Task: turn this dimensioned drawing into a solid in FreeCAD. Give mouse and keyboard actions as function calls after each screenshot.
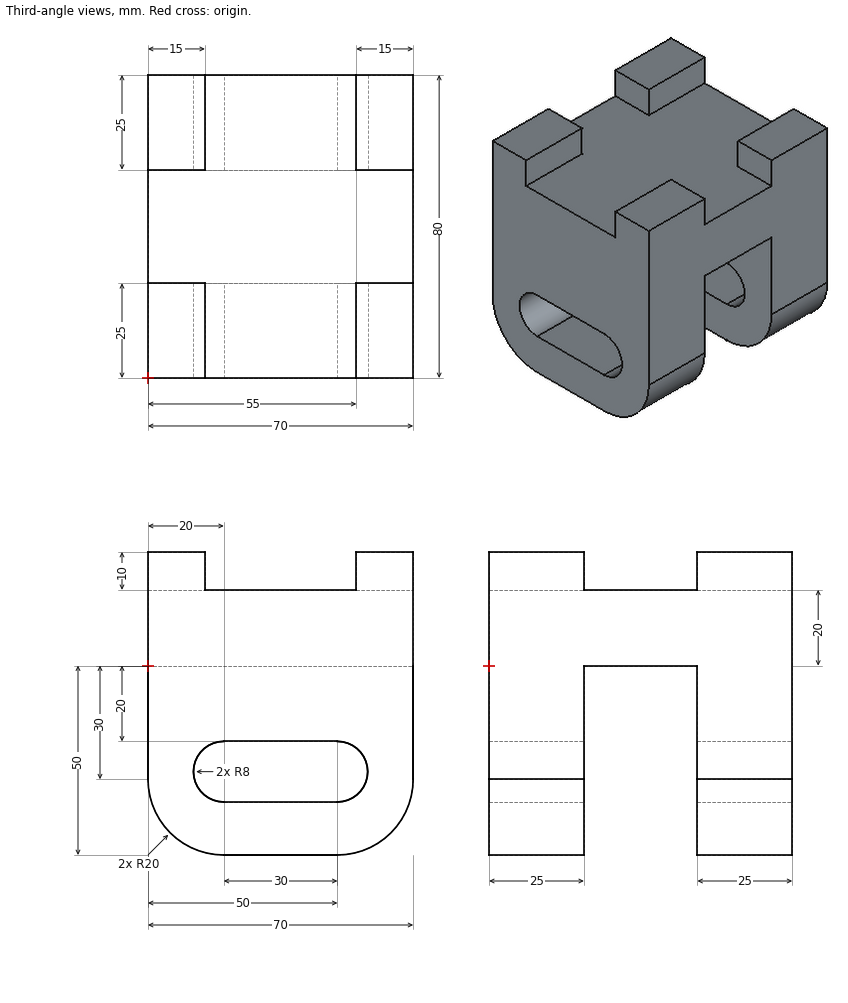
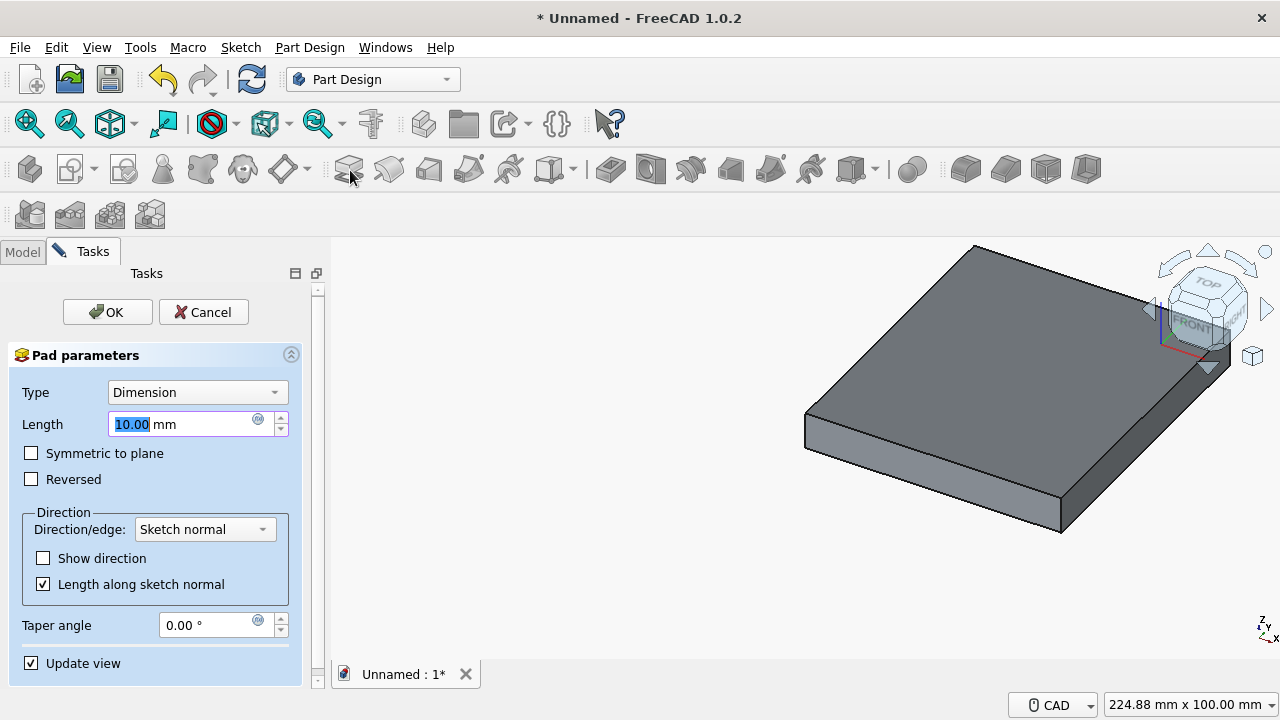
text(20)
key(Tab)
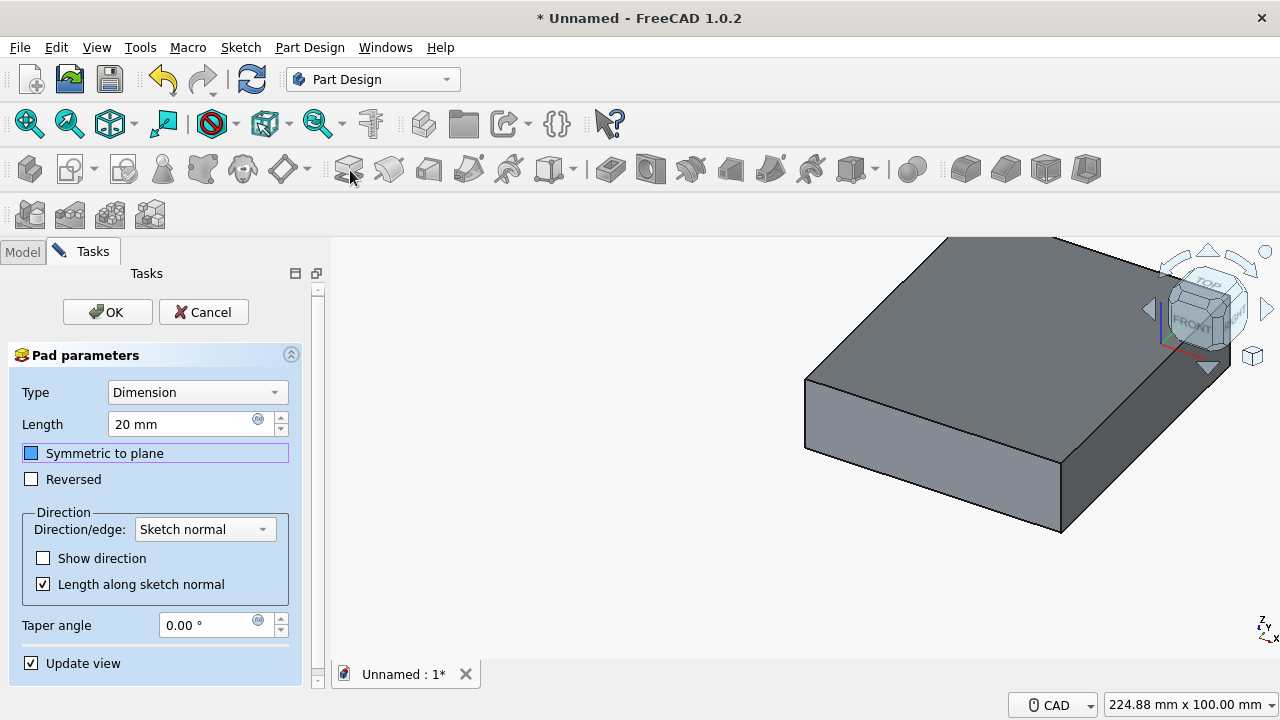
click(108, 312)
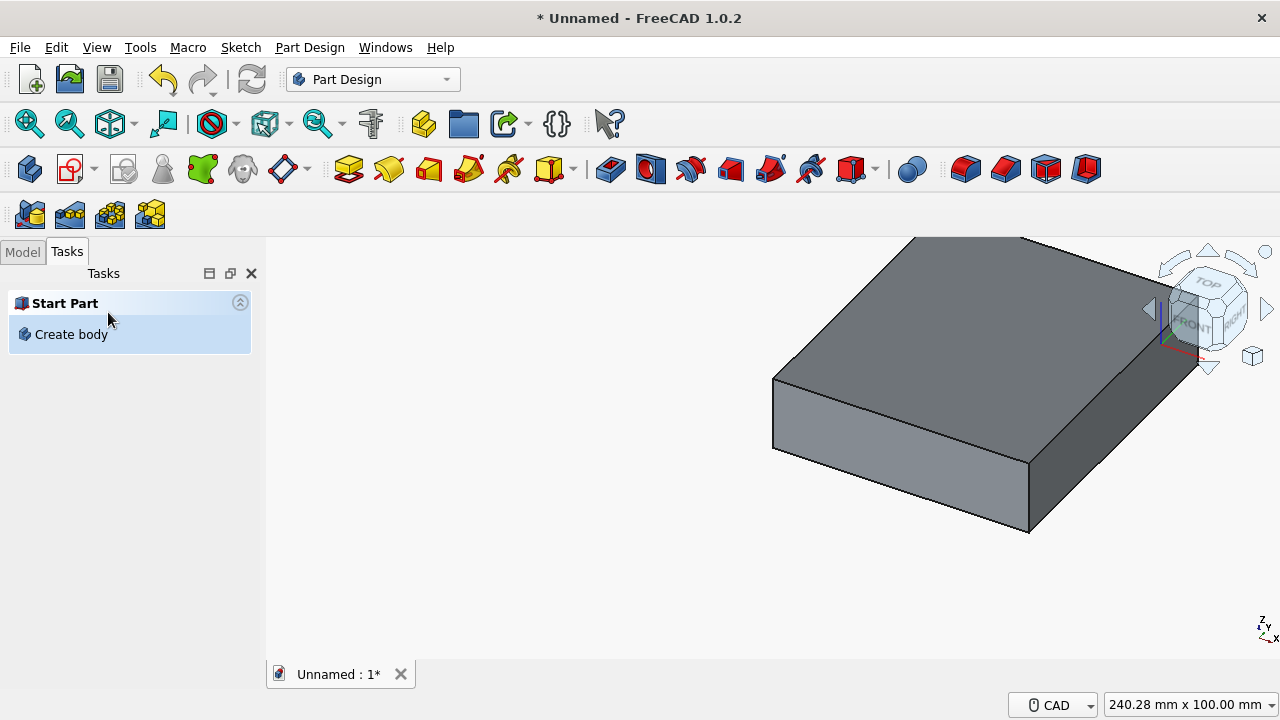
click(30, 124)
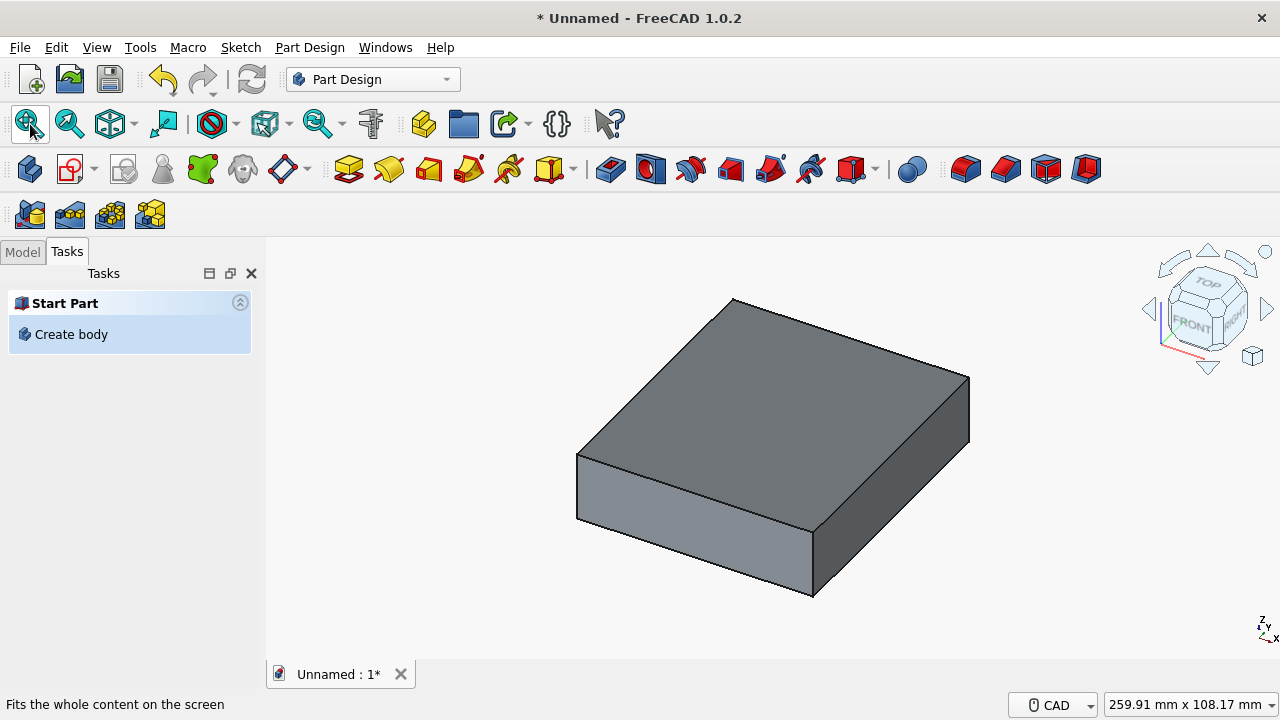
click(773, 415)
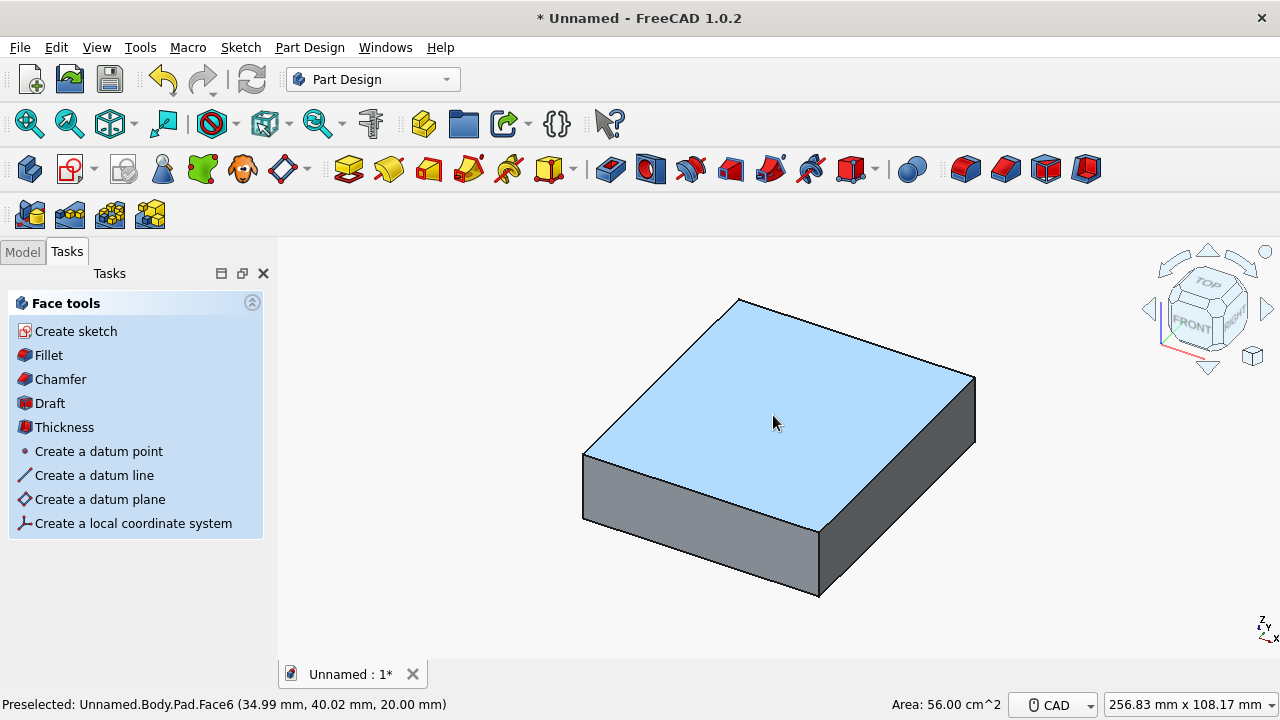
click(70, 170)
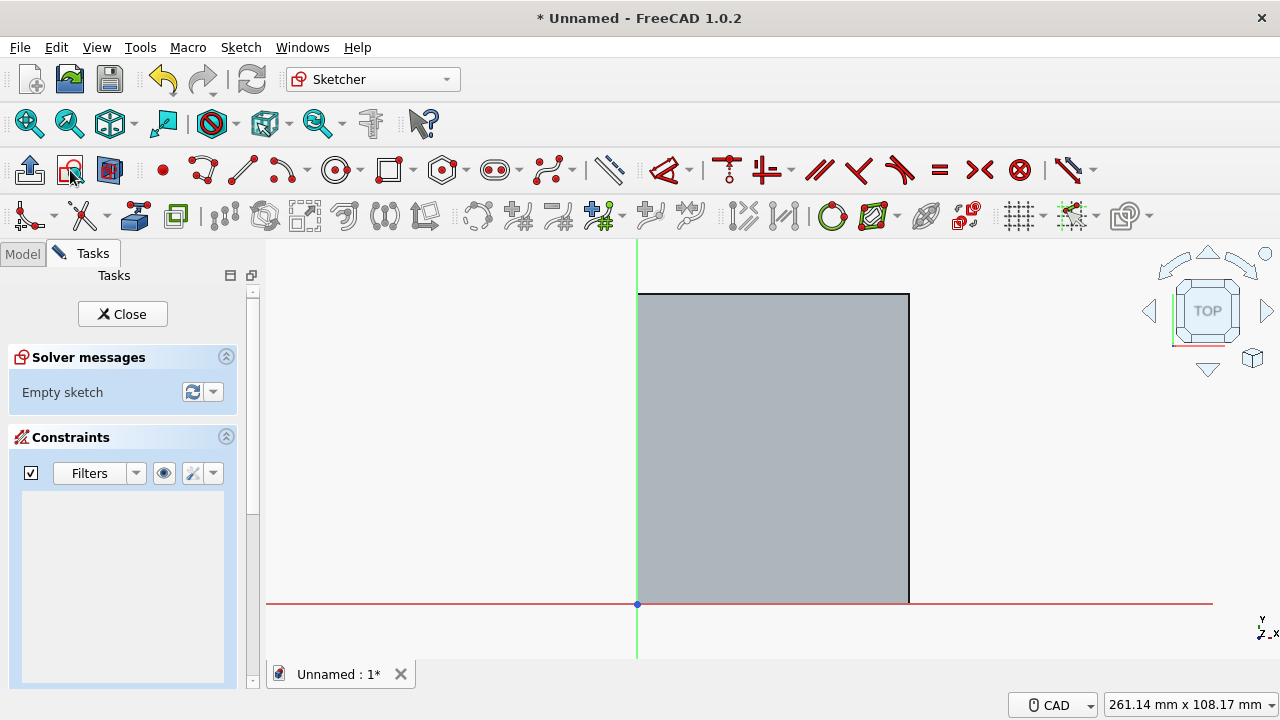
click(390, 170)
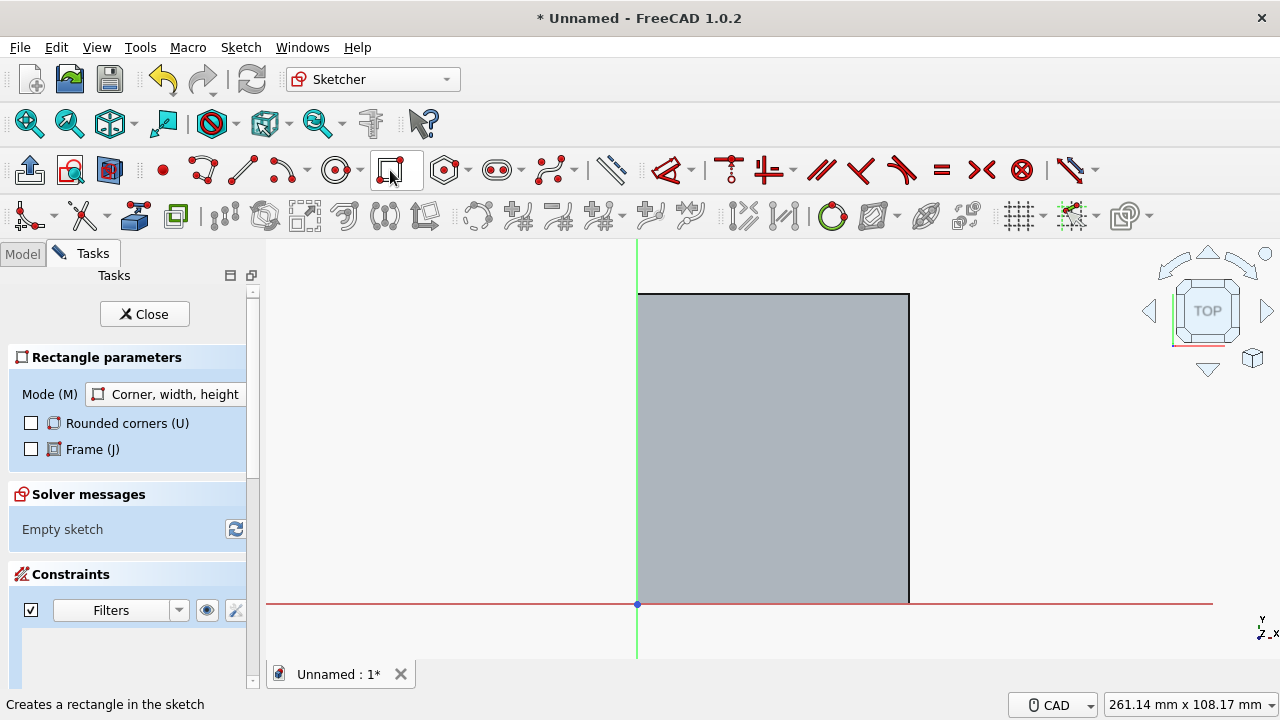
click(637, 294)
move(695, 391)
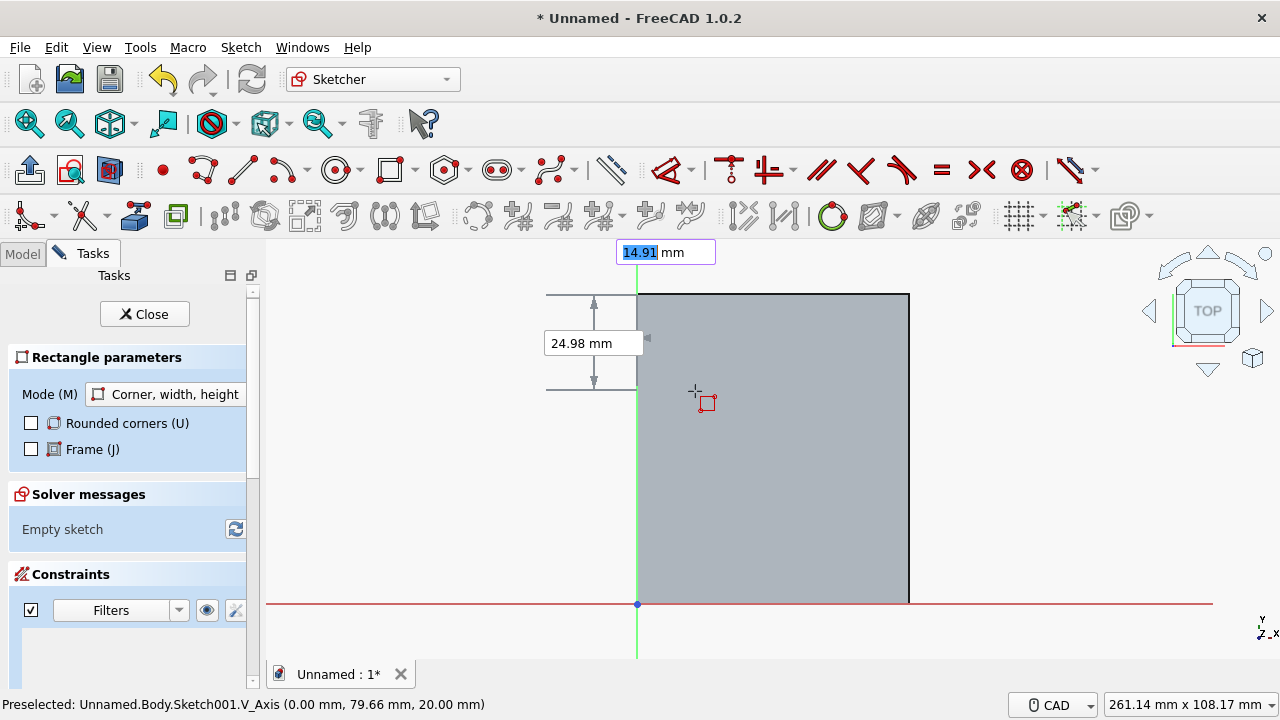
text(15)
key(Tab)
text(25)
key(Return)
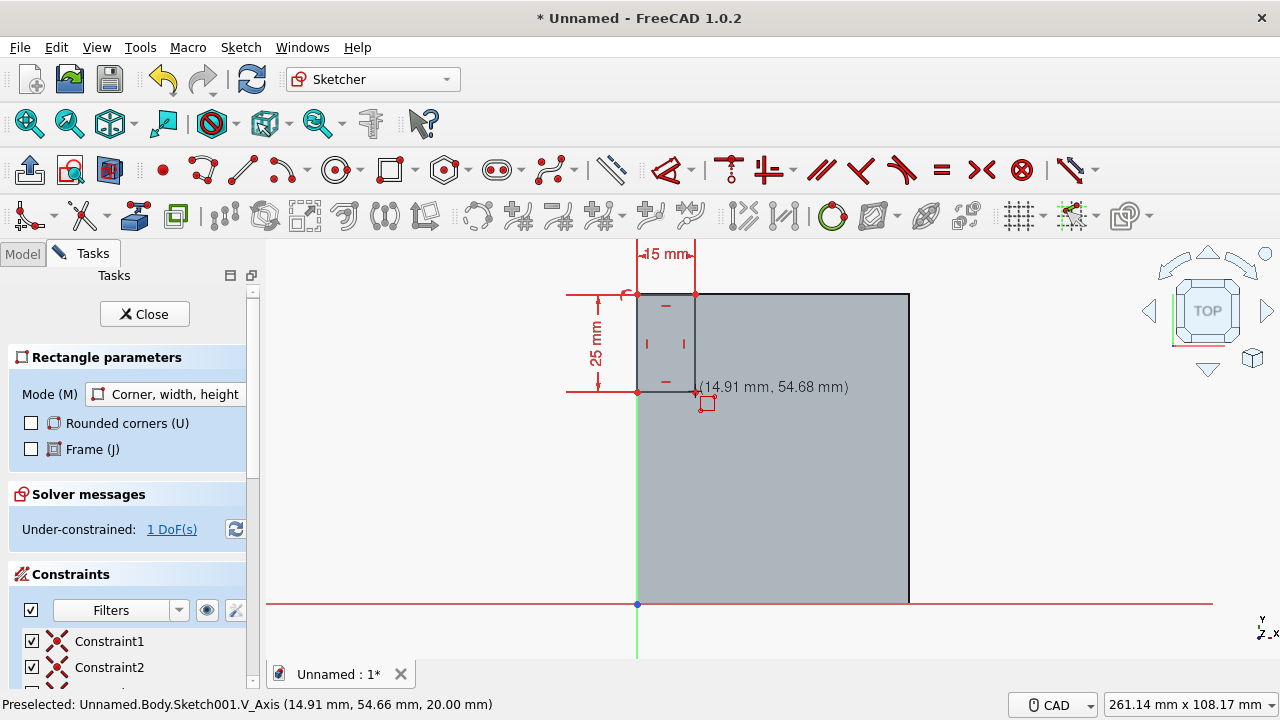
click(851, 294)
move(909, 391)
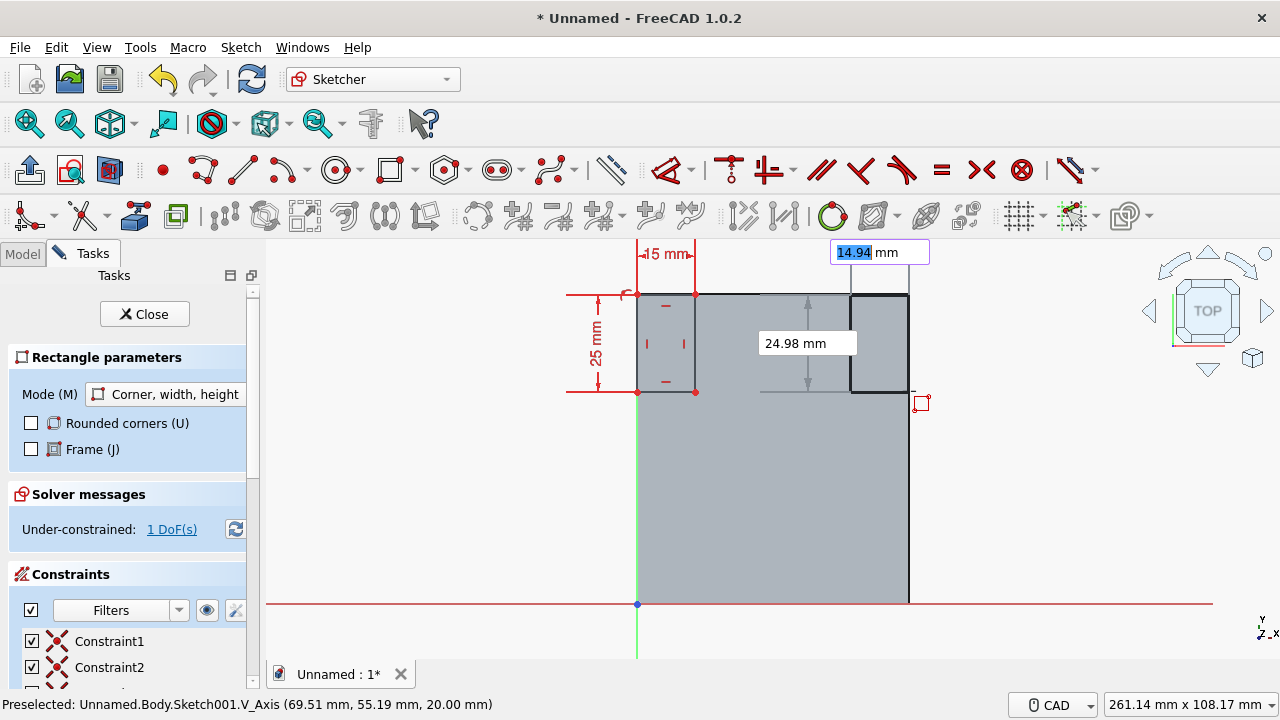
text(15)
key(Tab)
text(25)
key(Return)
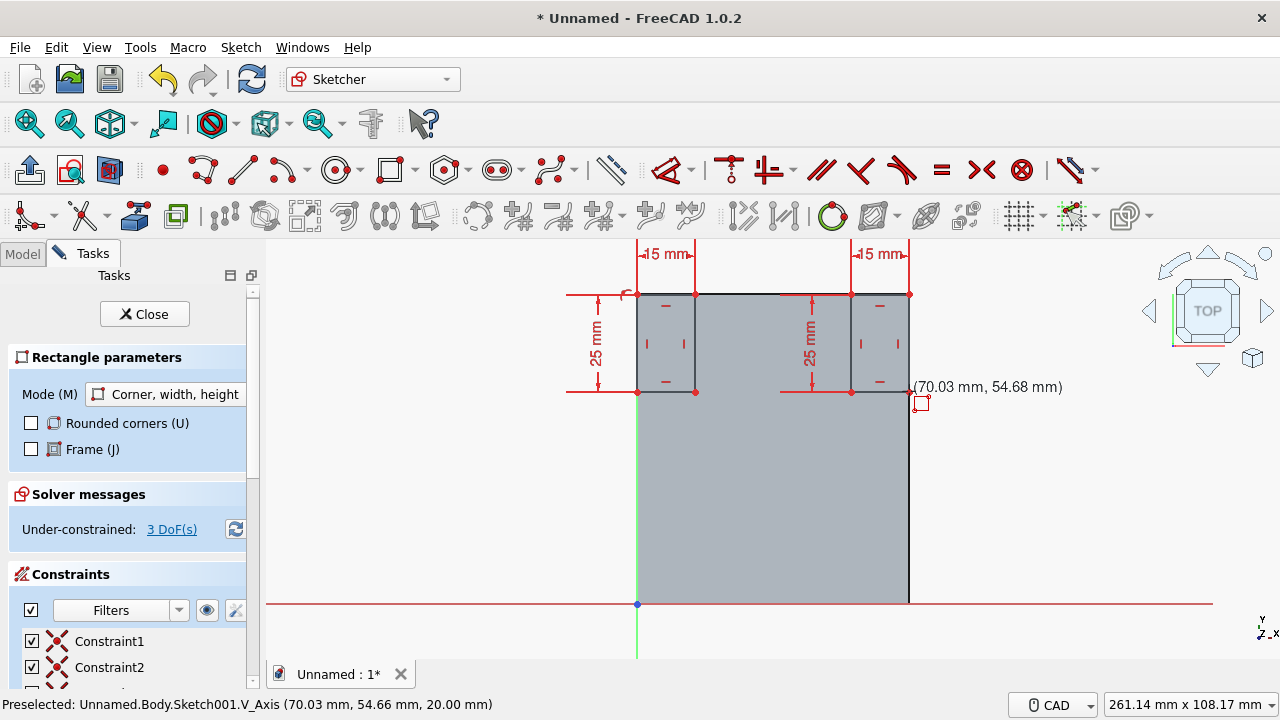
click(637, 604)
move(695, 507)